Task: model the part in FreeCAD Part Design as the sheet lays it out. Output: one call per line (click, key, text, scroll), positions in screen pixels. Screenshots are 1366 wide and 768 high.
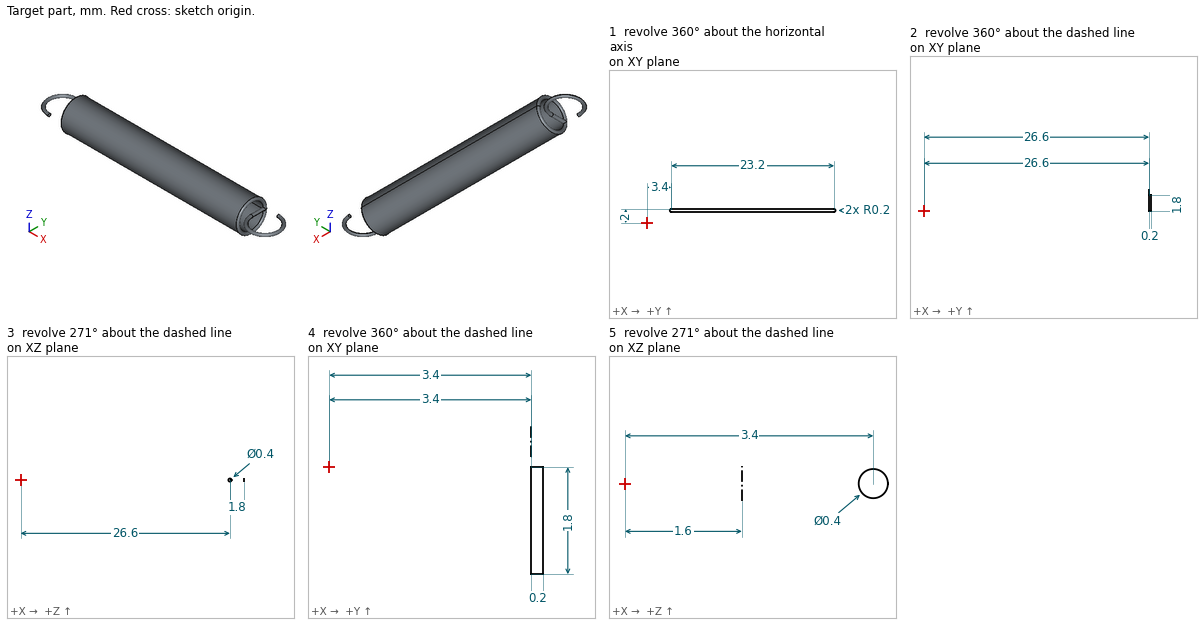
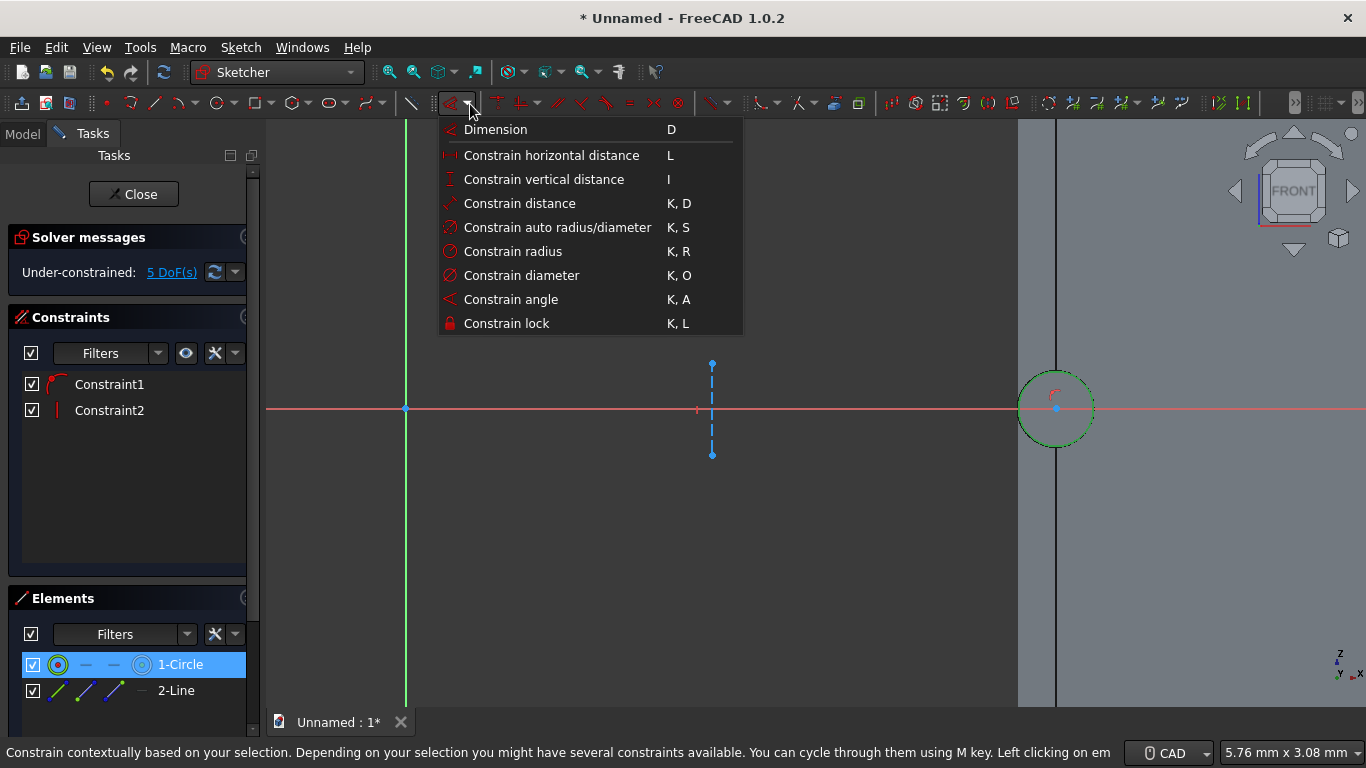
click(591, 275)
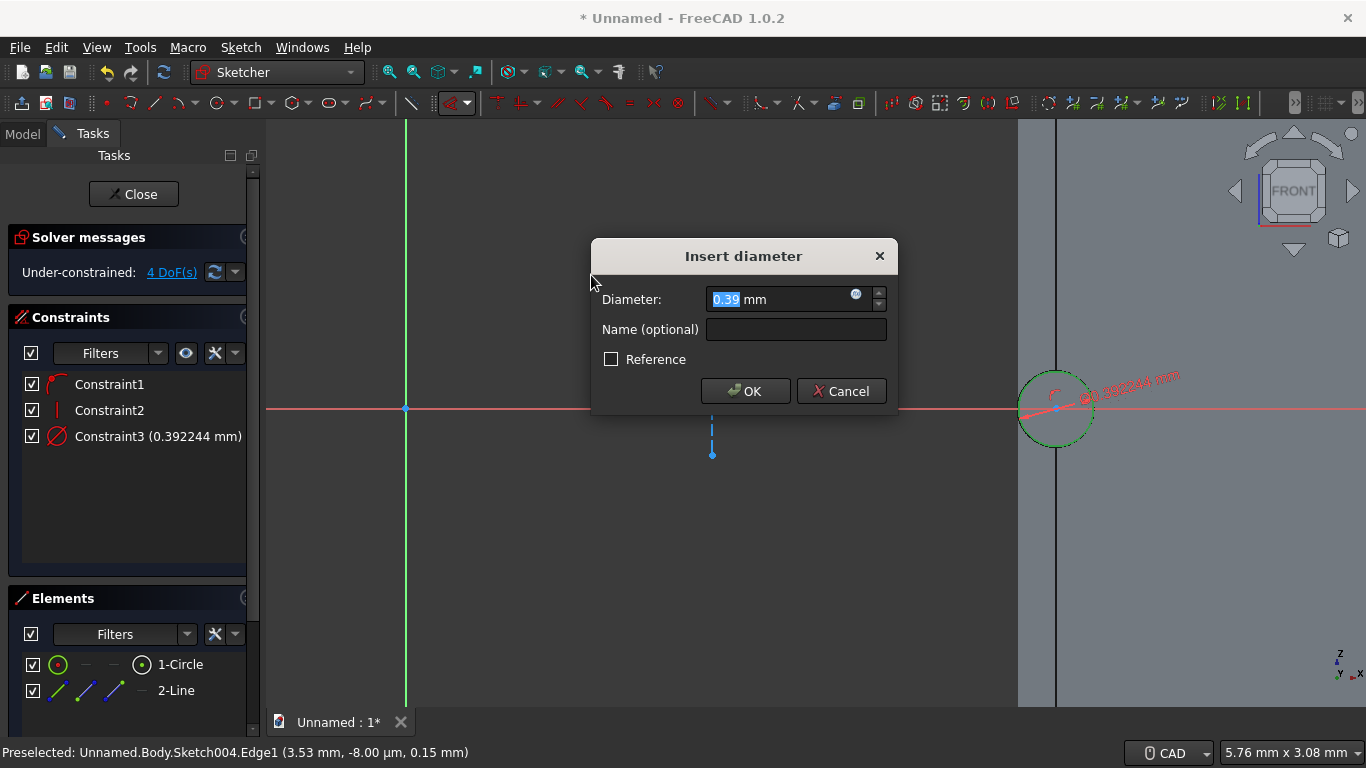
text(0.4)
key(Return)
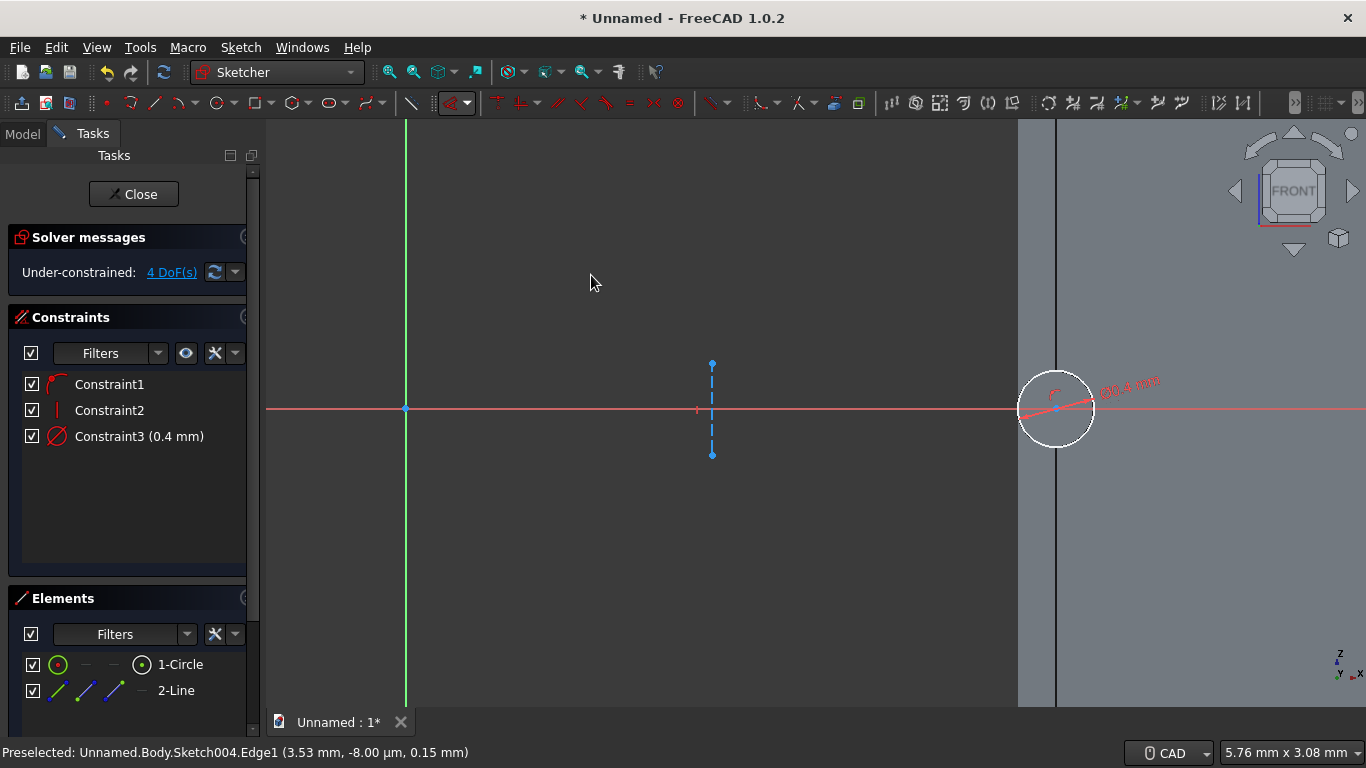
click(1056, 409)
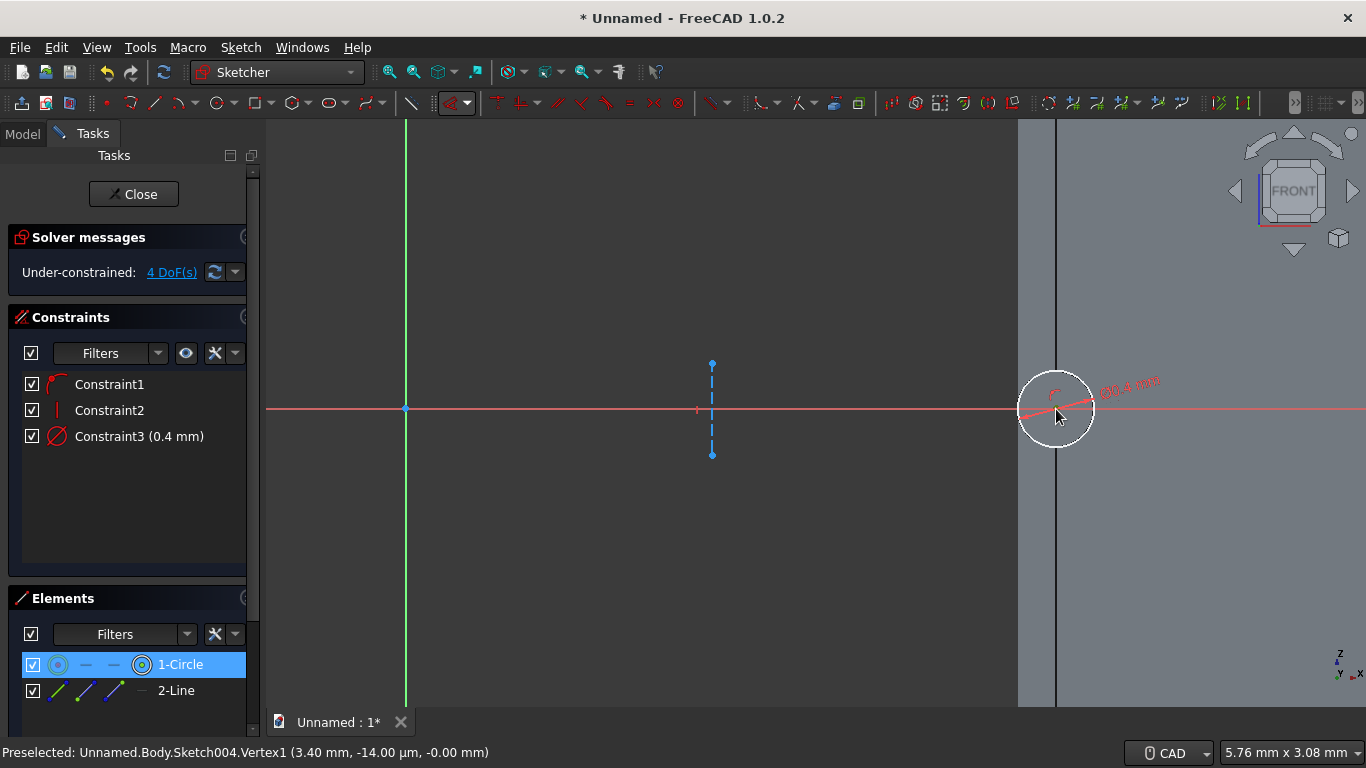
click(470, 104)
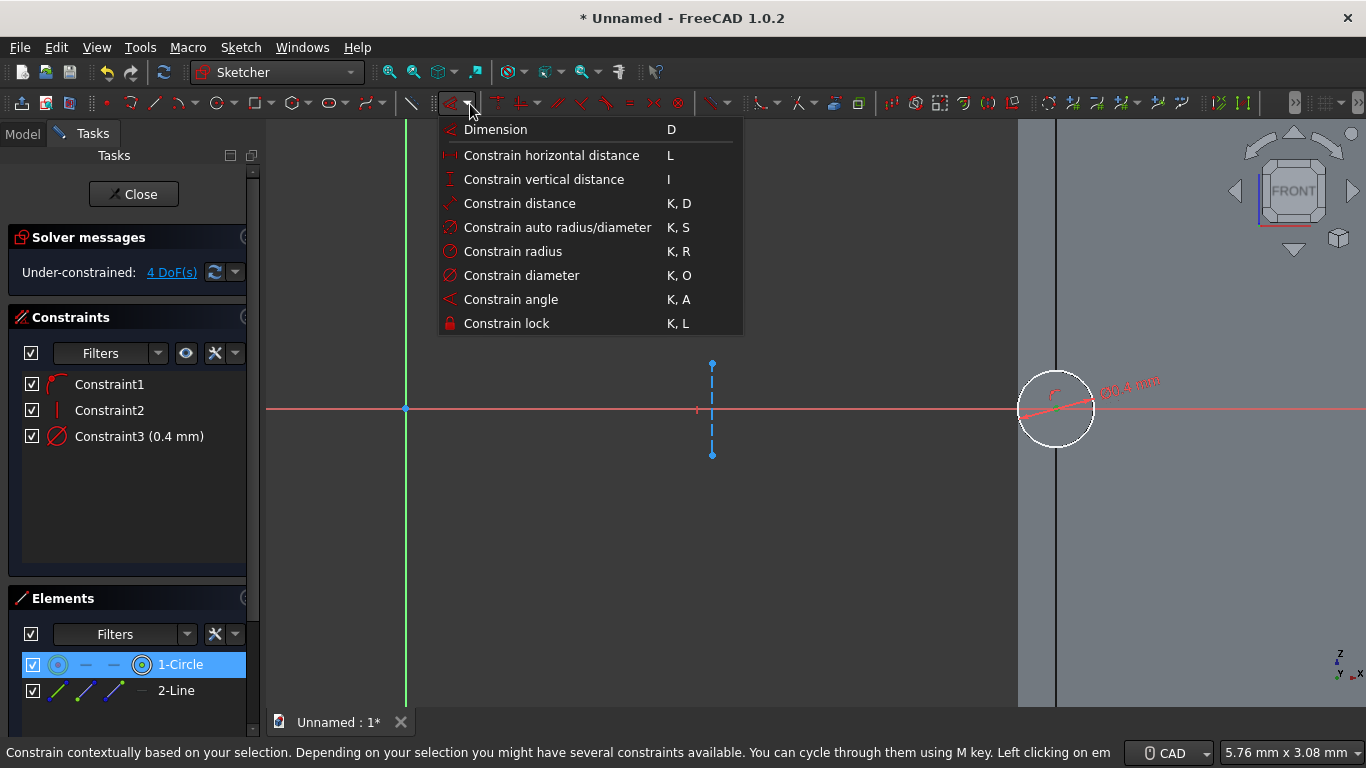
click(591, 155)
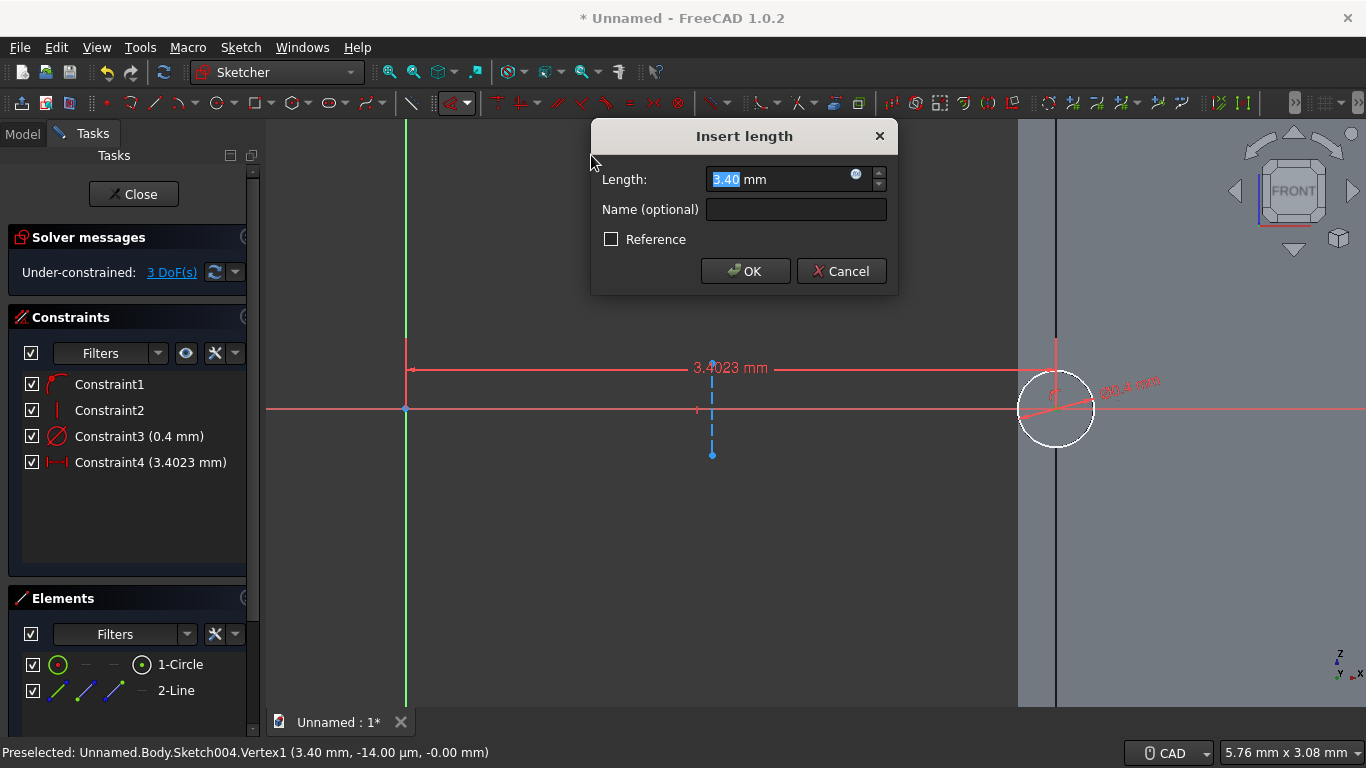
text(3.4)
key(Return)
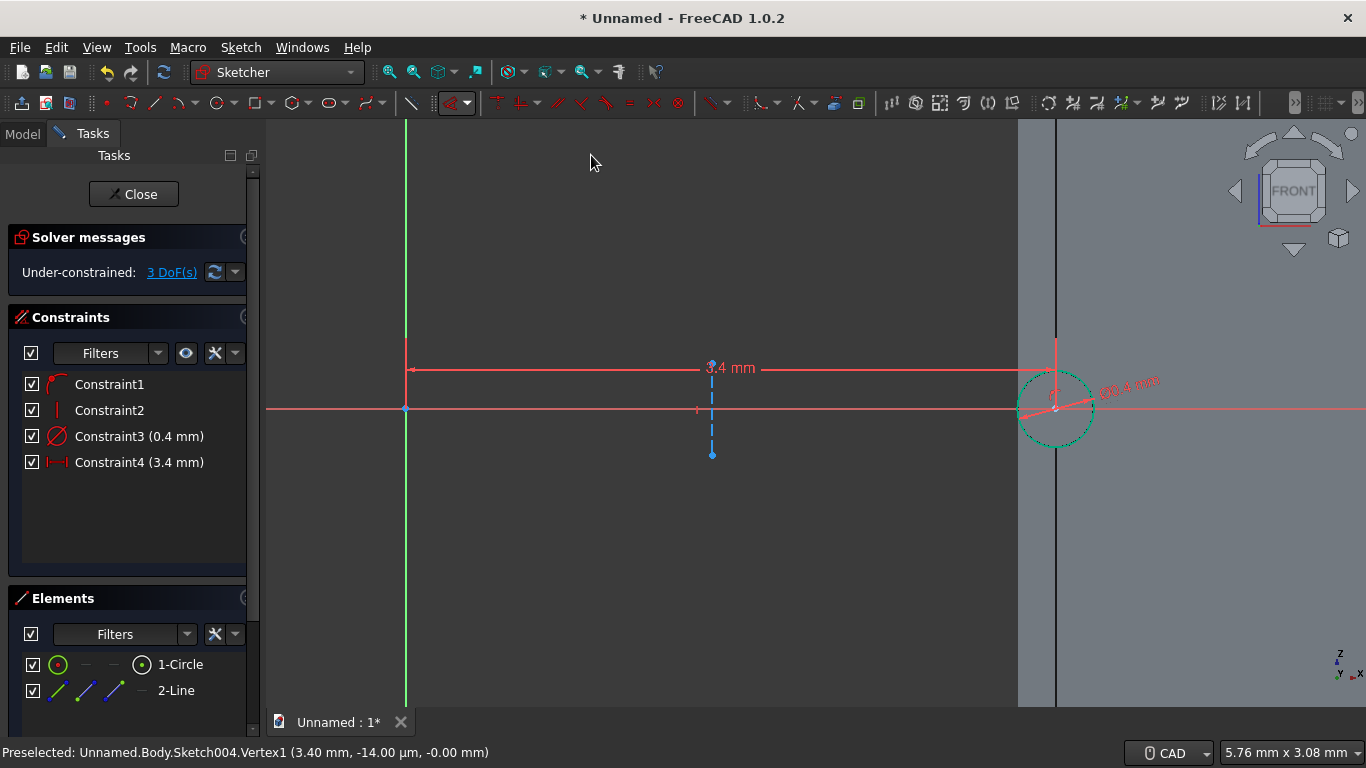
click(712, 456)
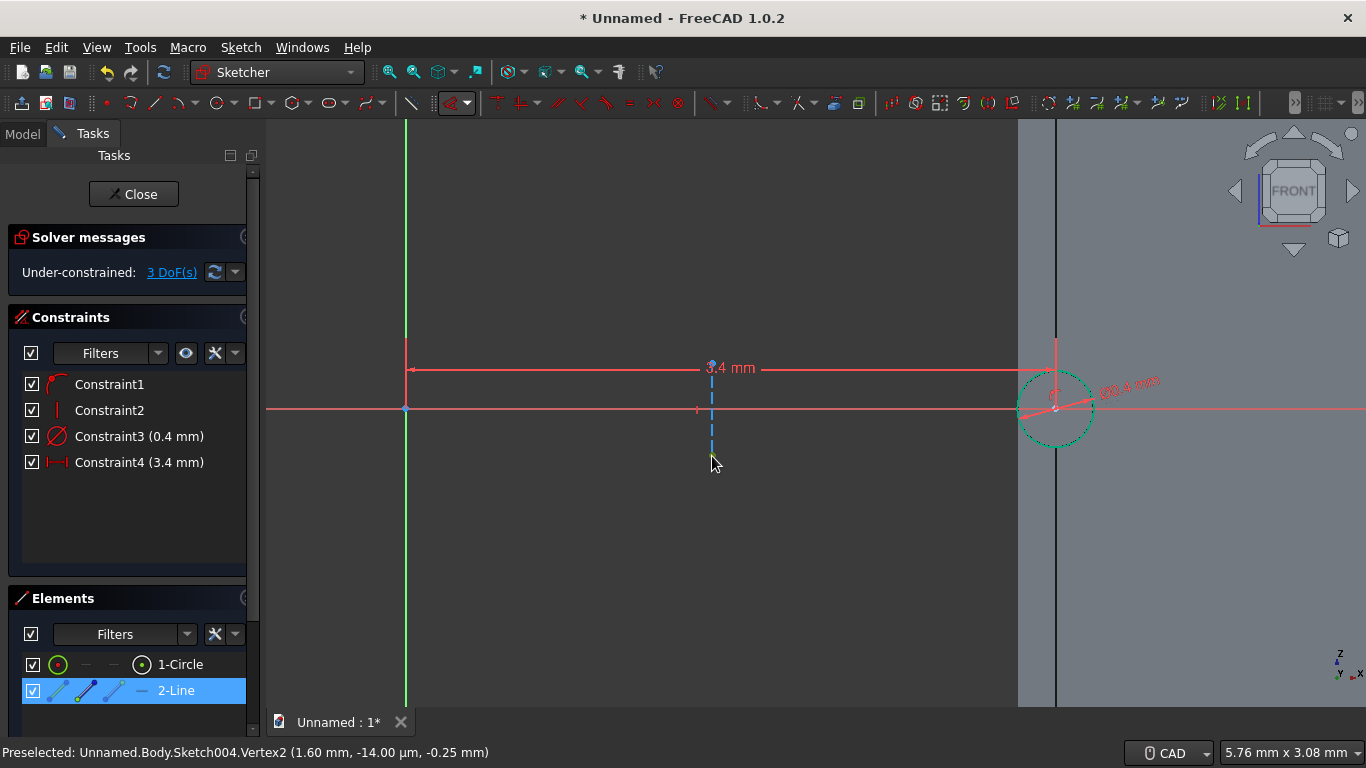
click(470, 104)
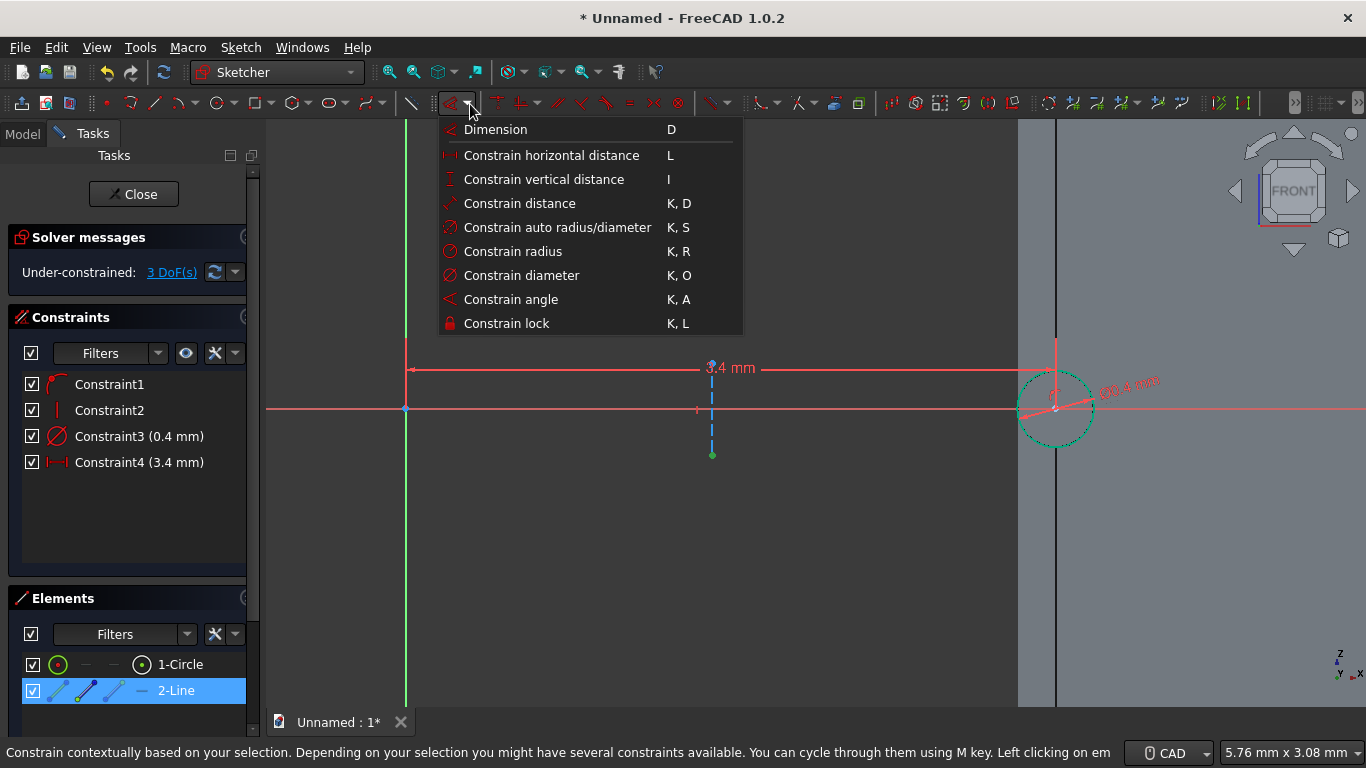
click(591, 155)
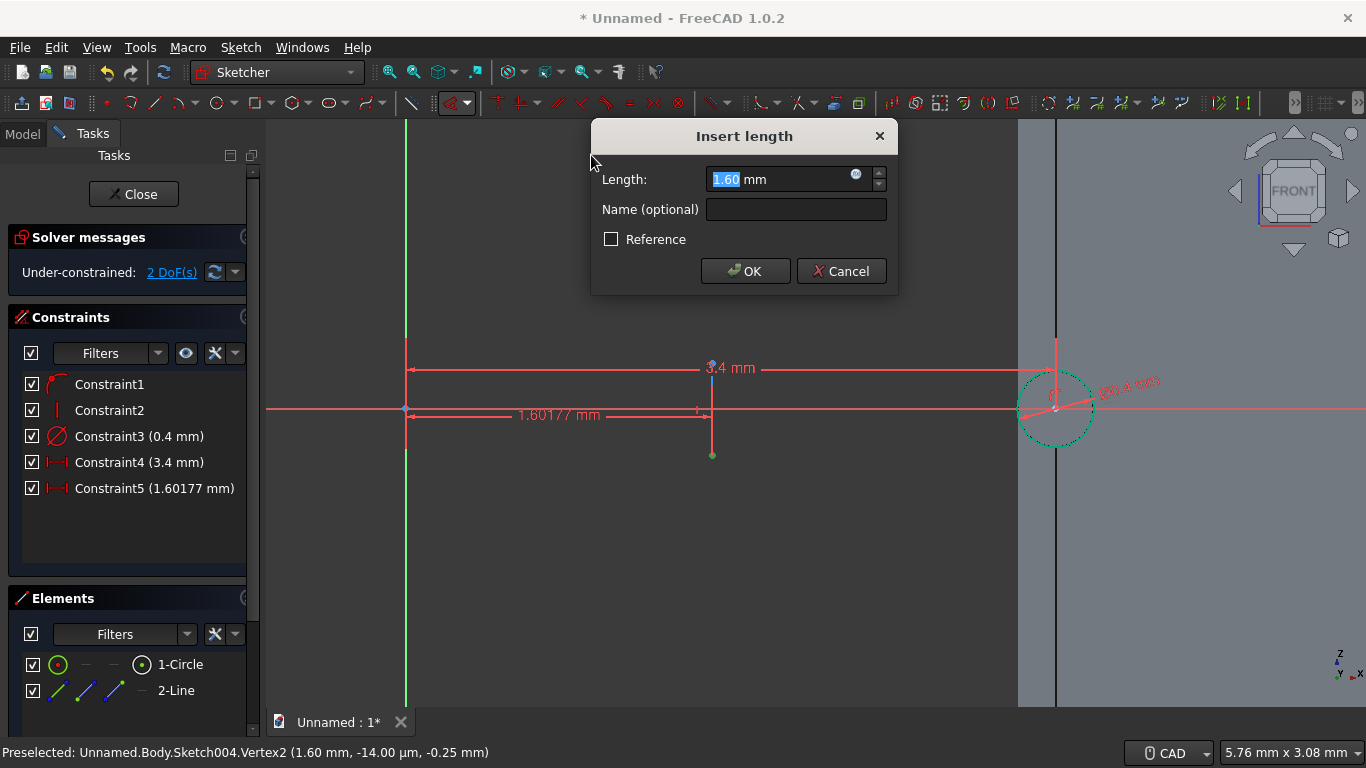
text(1.6)
key(Return)